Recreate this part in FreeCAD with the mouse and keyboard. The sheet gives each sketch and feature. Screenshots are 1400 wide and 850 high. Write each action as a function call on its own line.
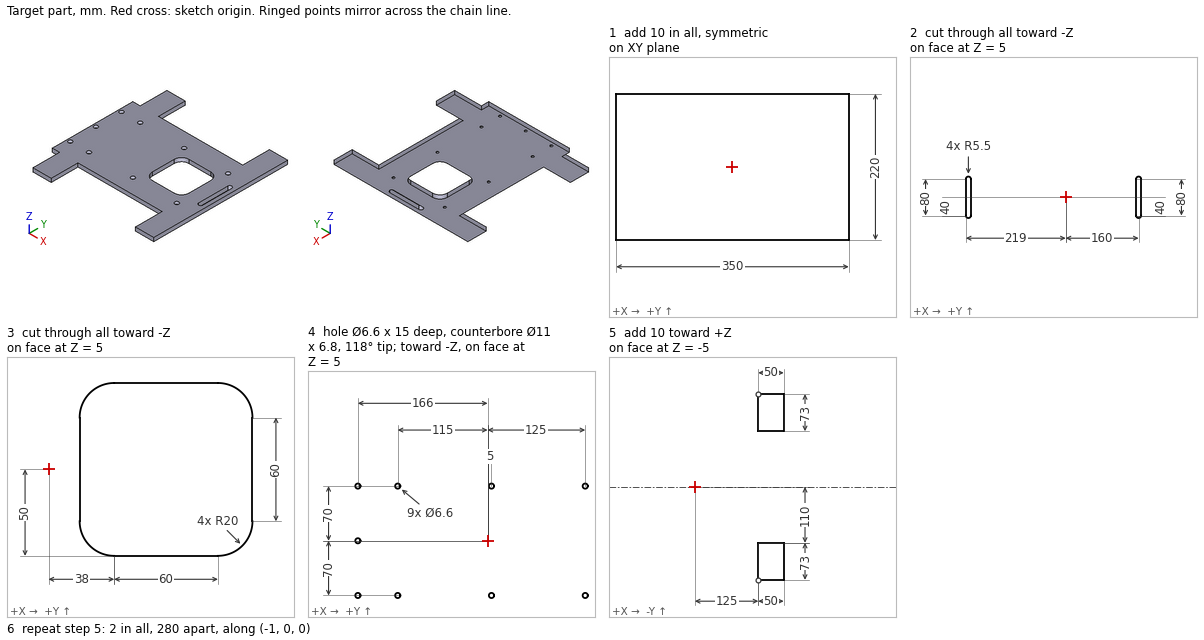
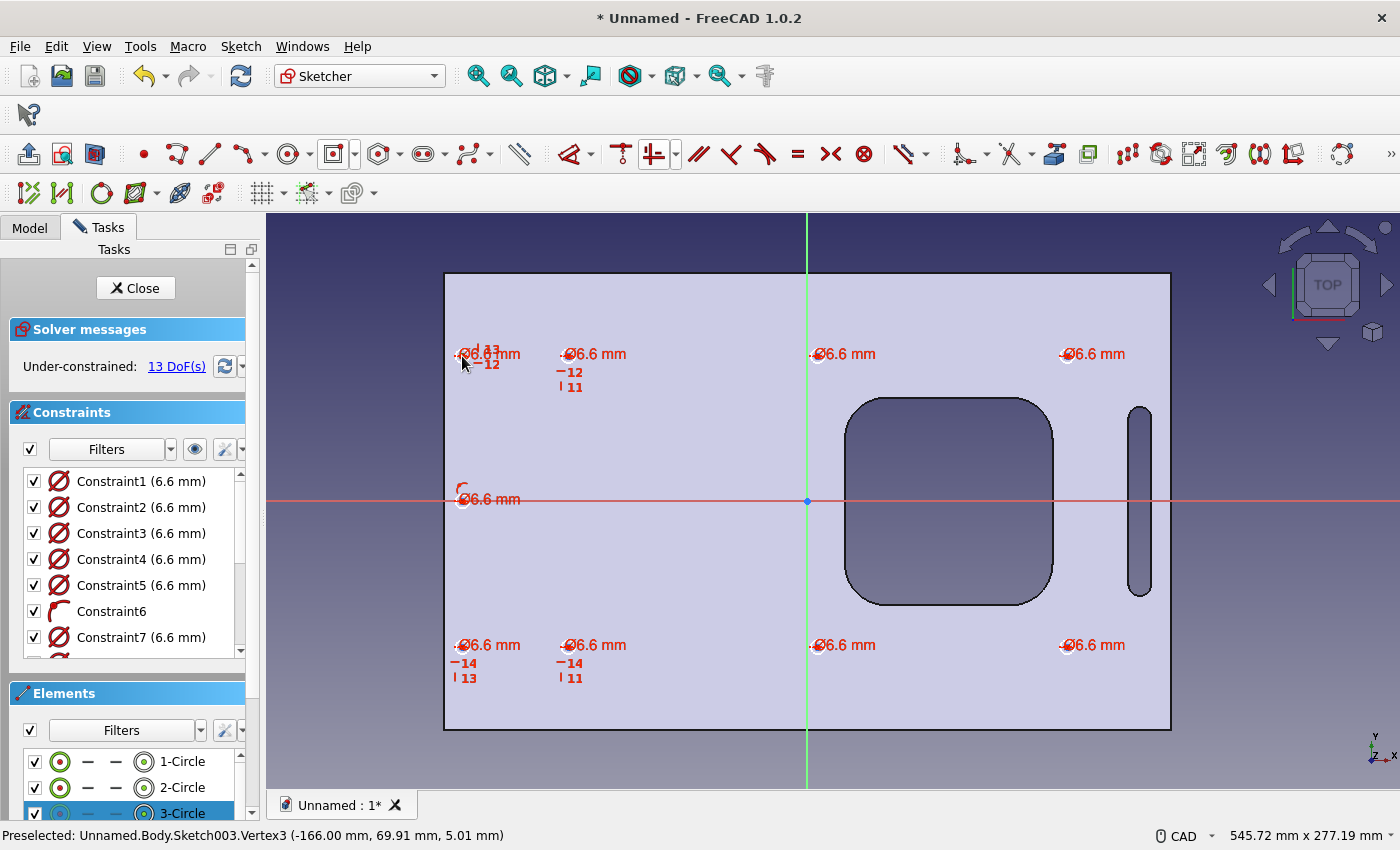
click(462, 501)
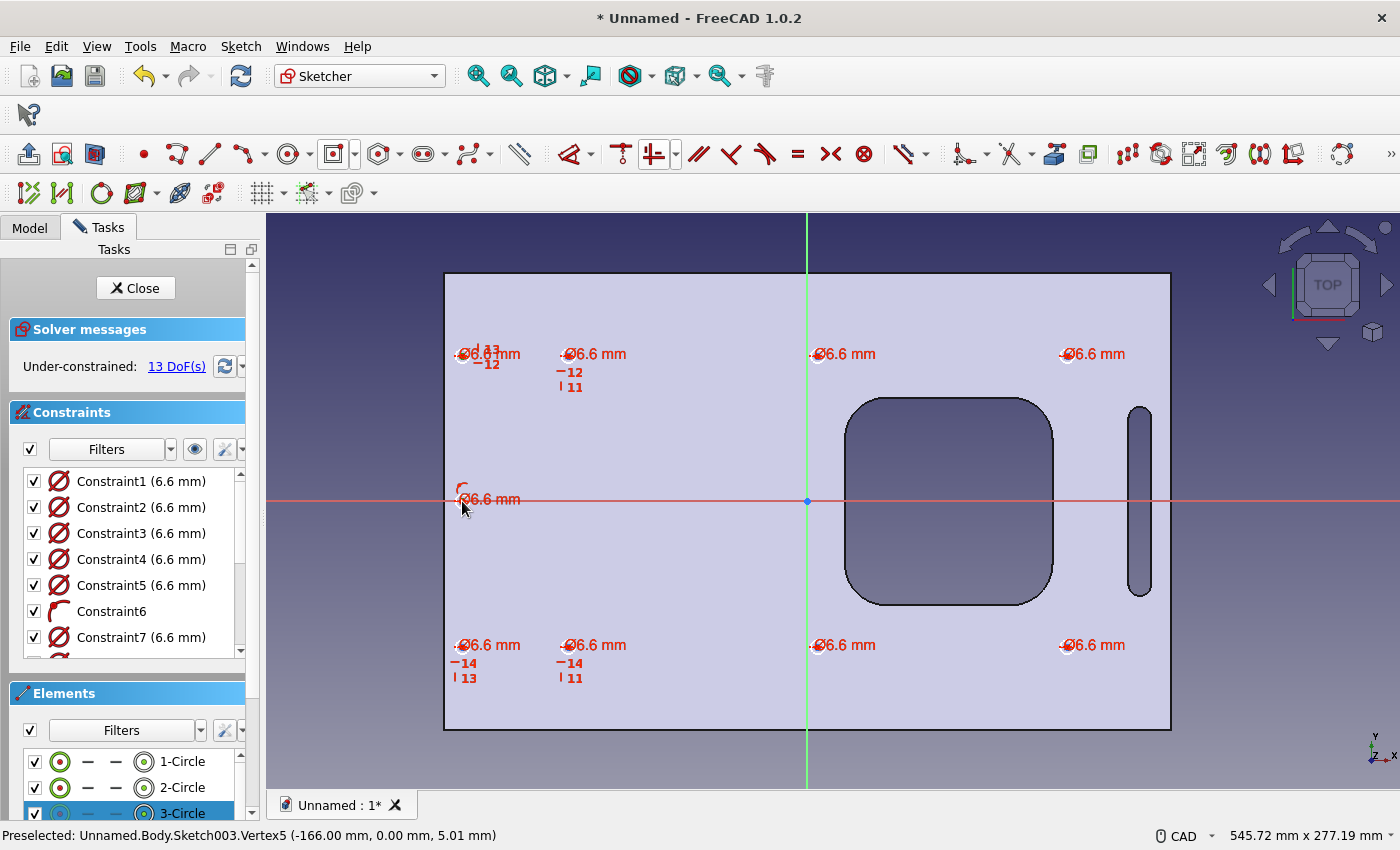
key(v)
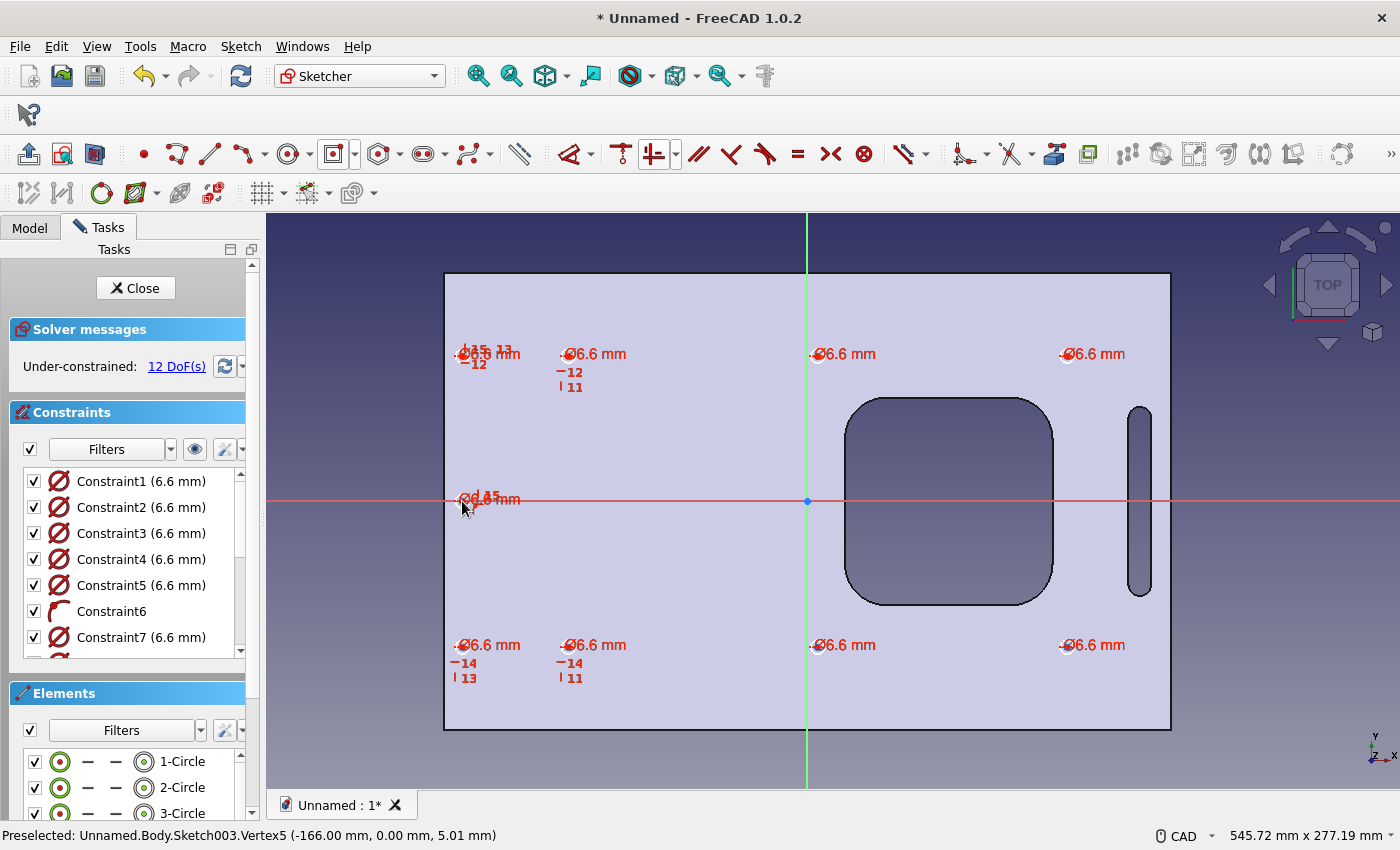
click(568, 356)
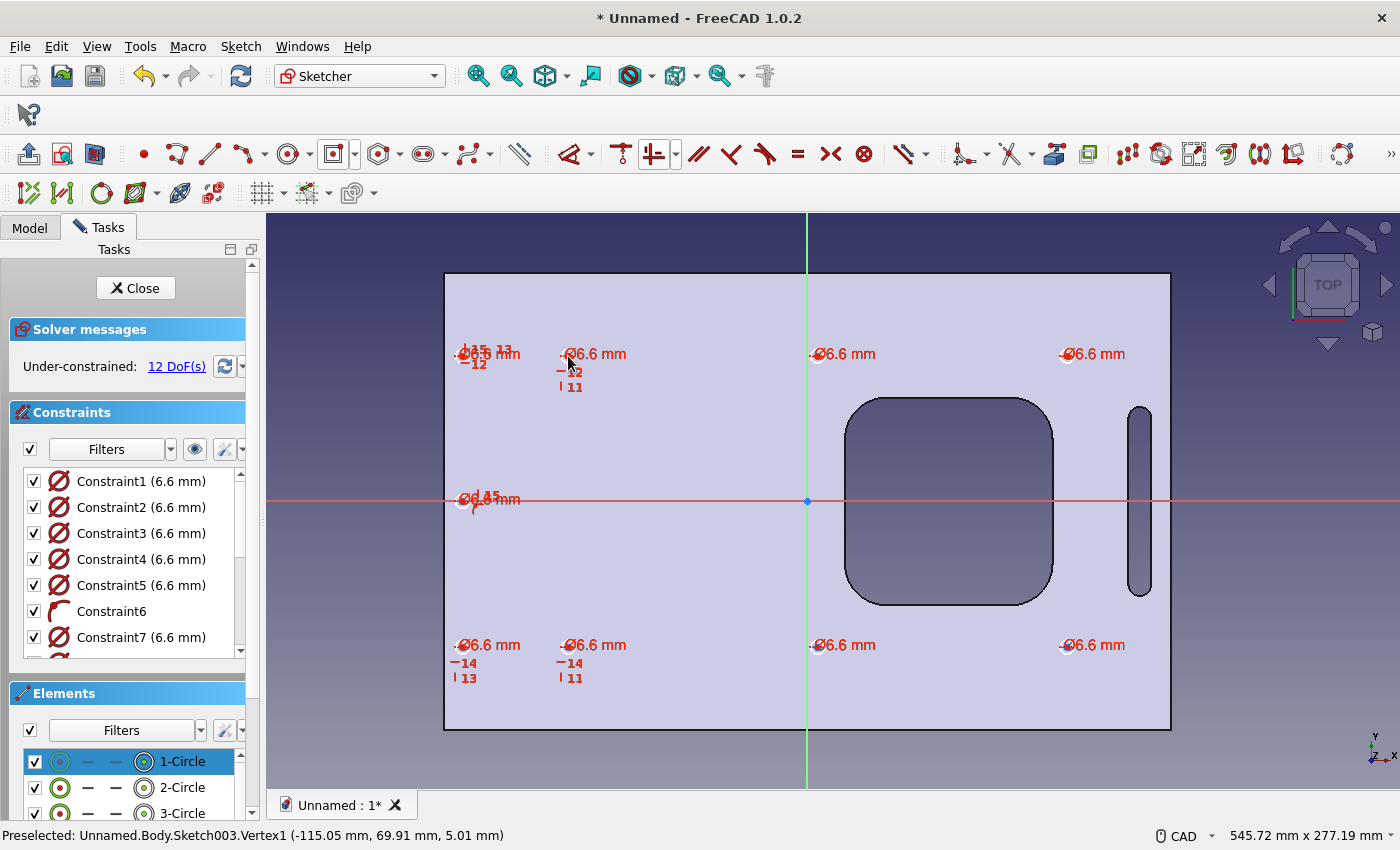
click(818, 356)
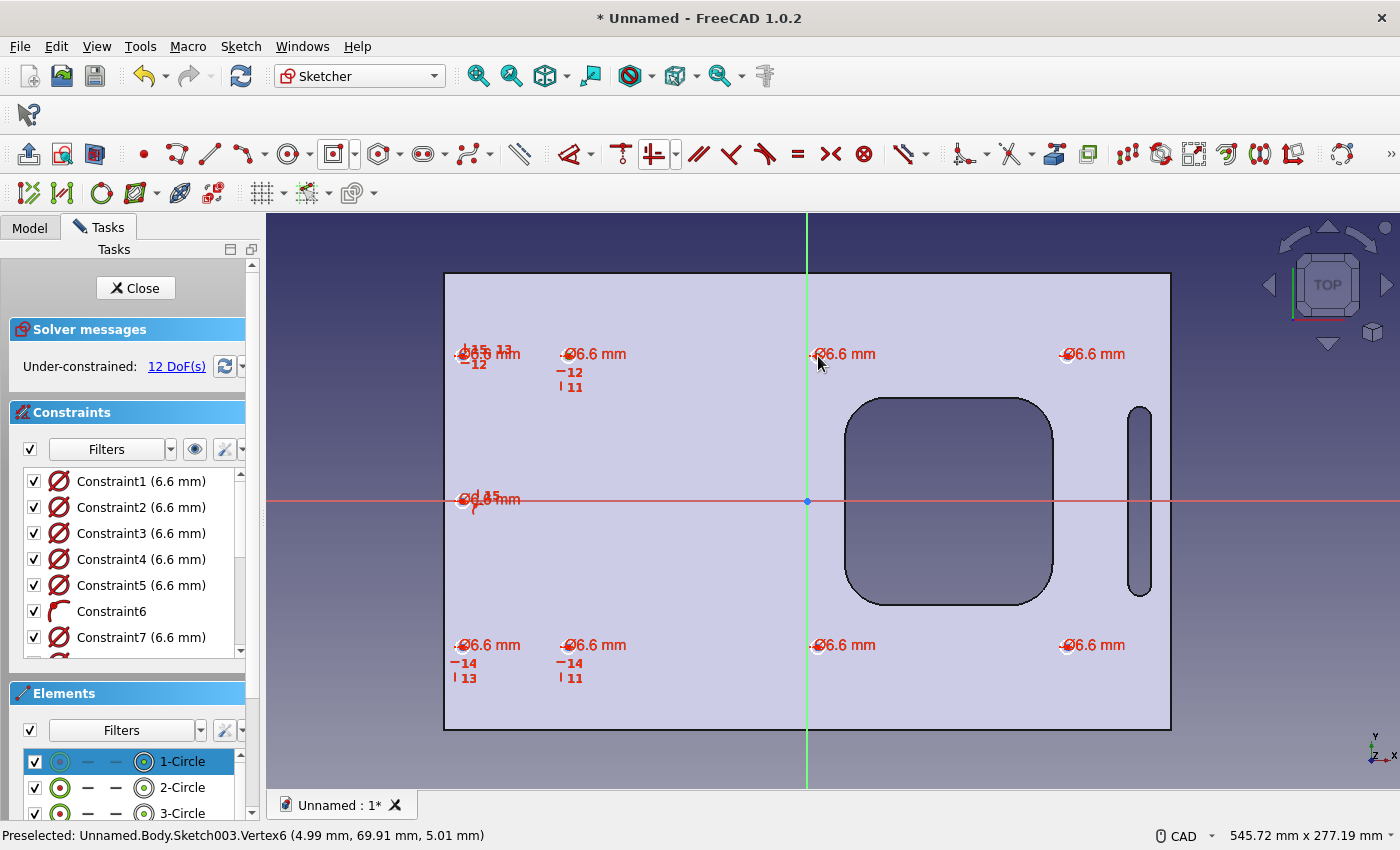
click(676, 154)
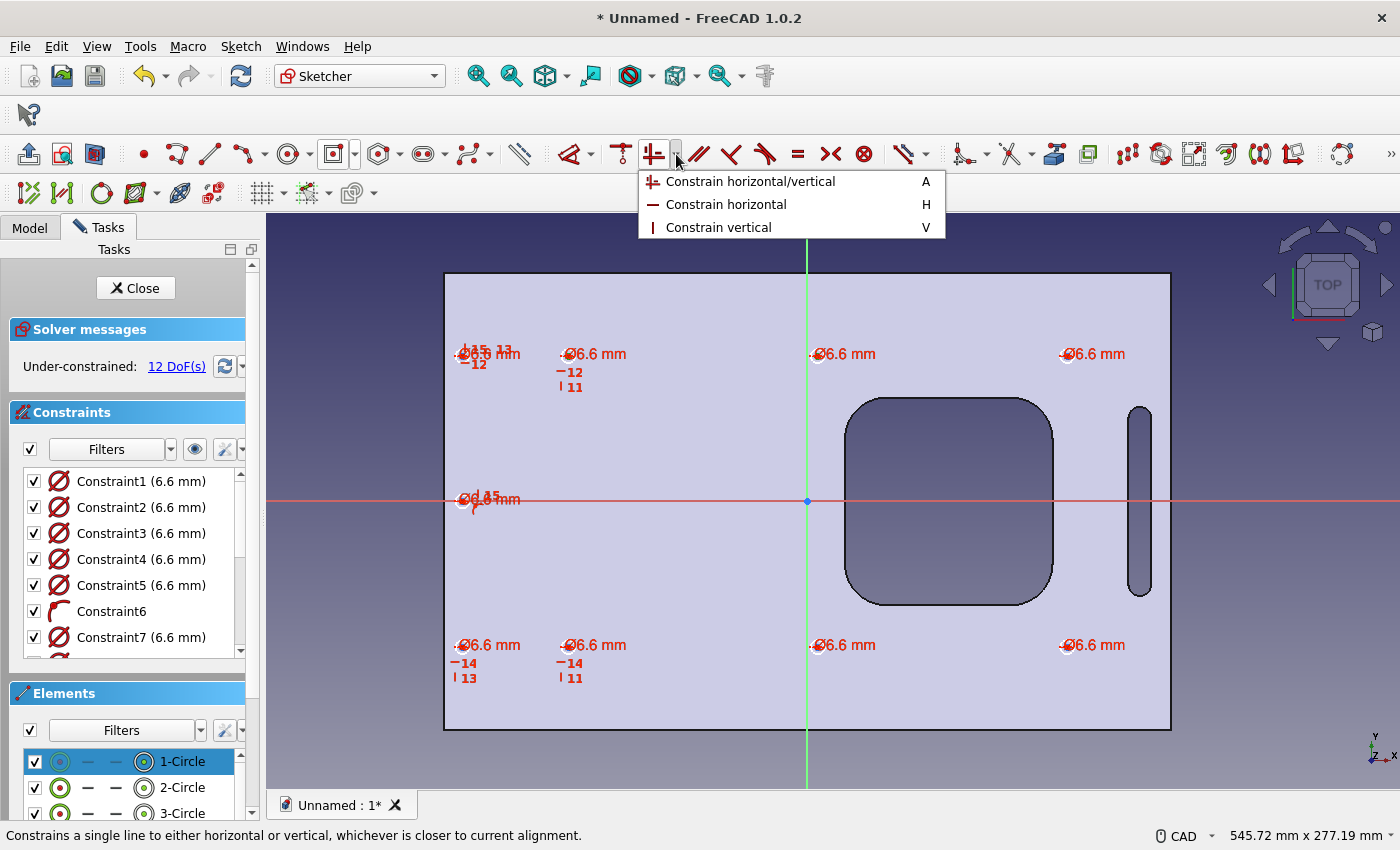
click(792, 204)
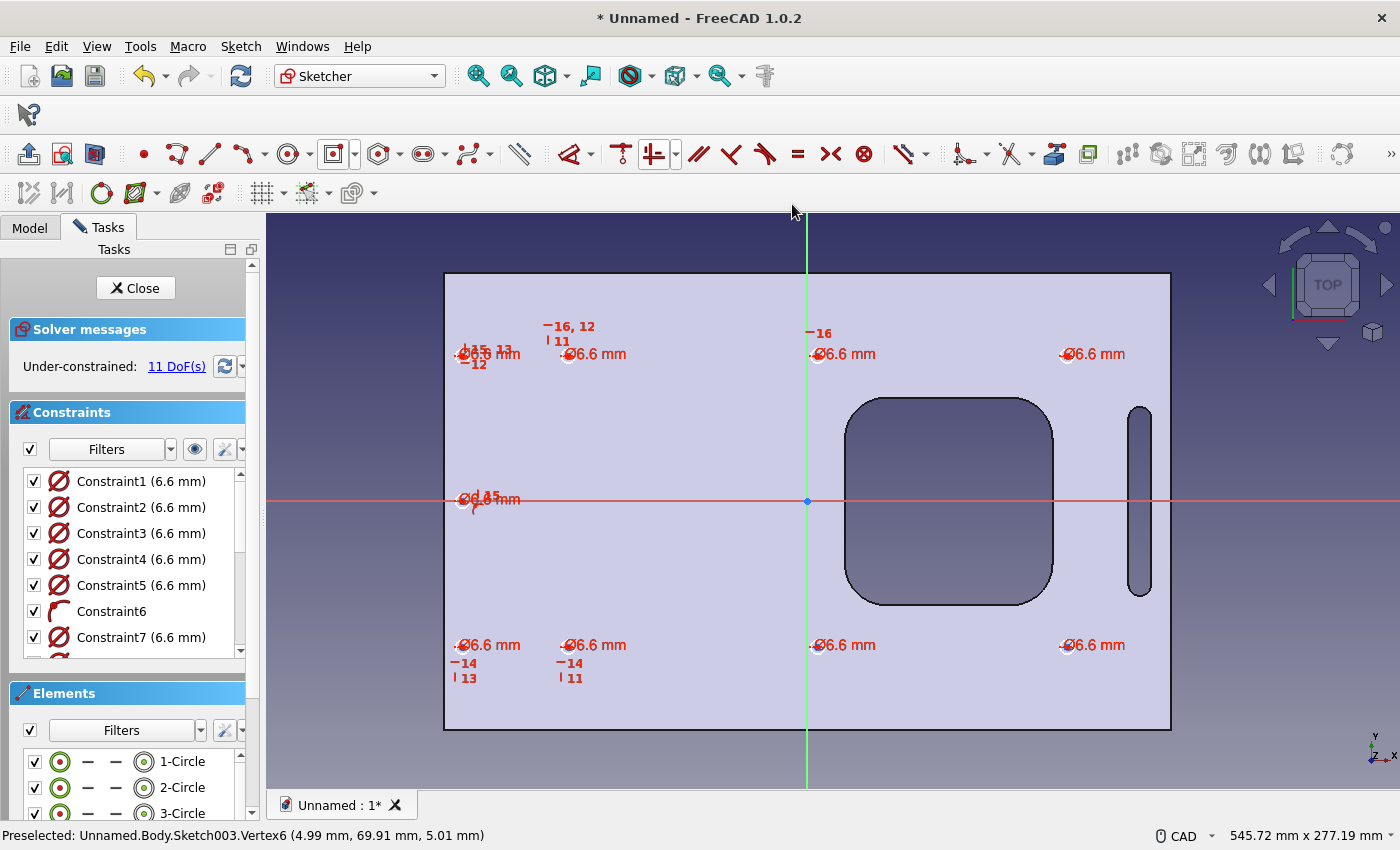
click(818, 356)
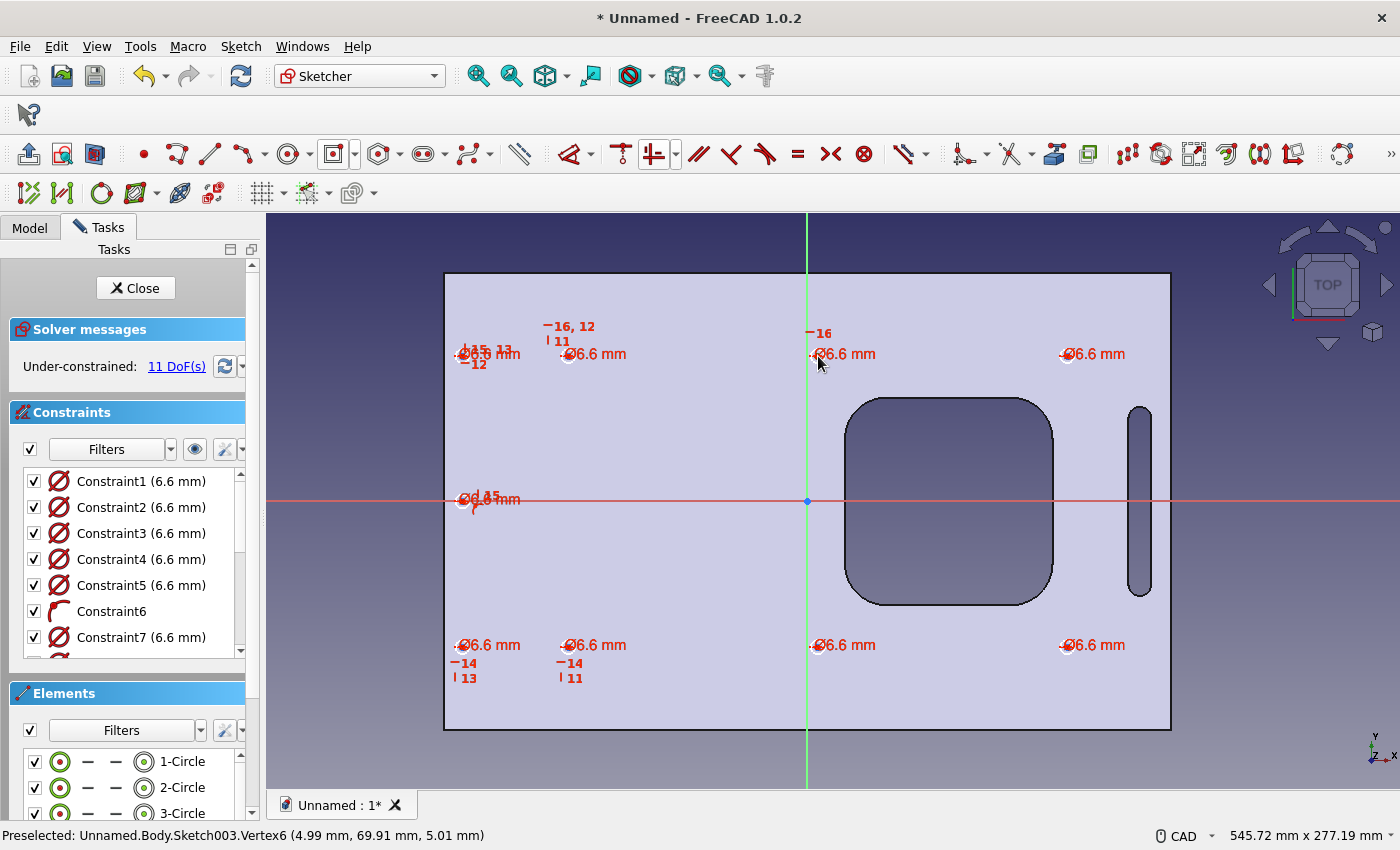
click(1067, 356)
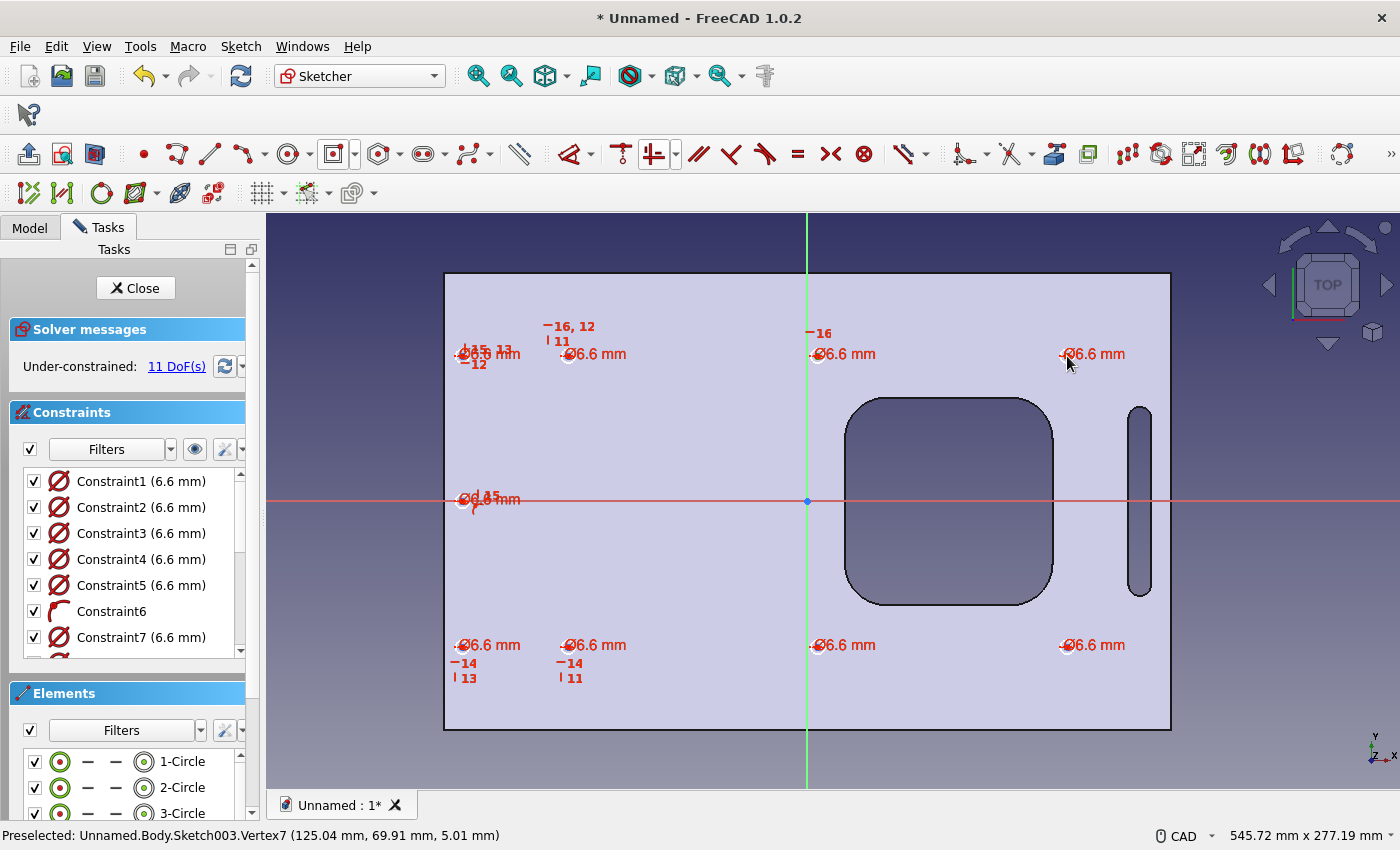
key(h)